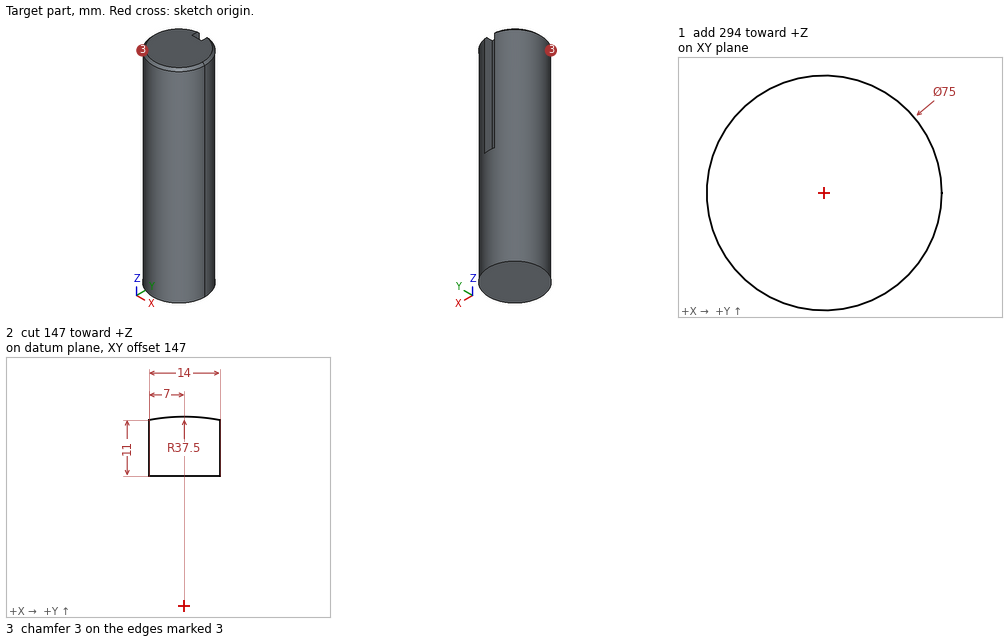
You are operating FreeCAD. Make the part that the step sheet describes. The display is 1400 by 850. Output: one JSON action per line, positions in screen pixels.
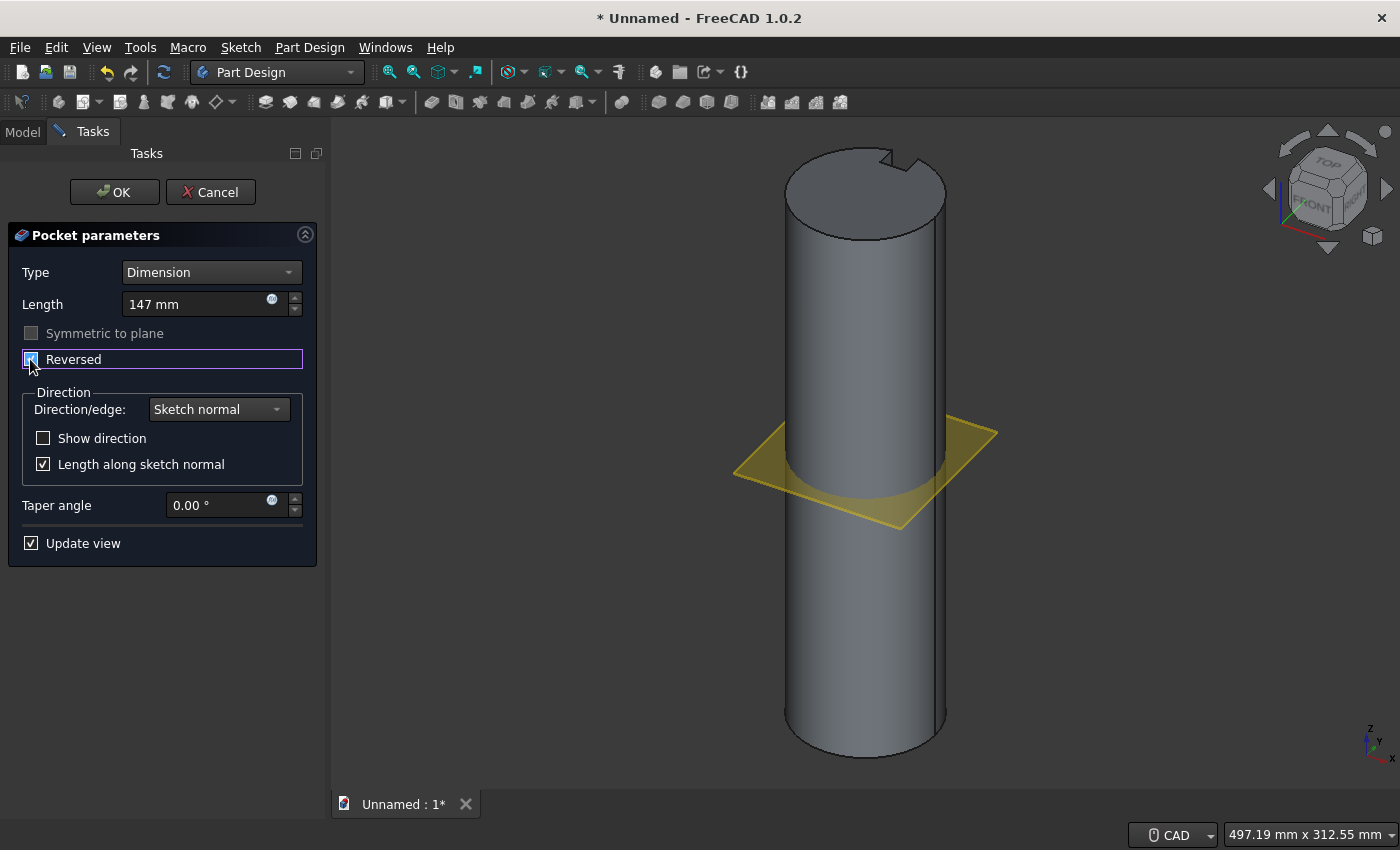
{"action": "left_click", "coordinate": [115, 192]}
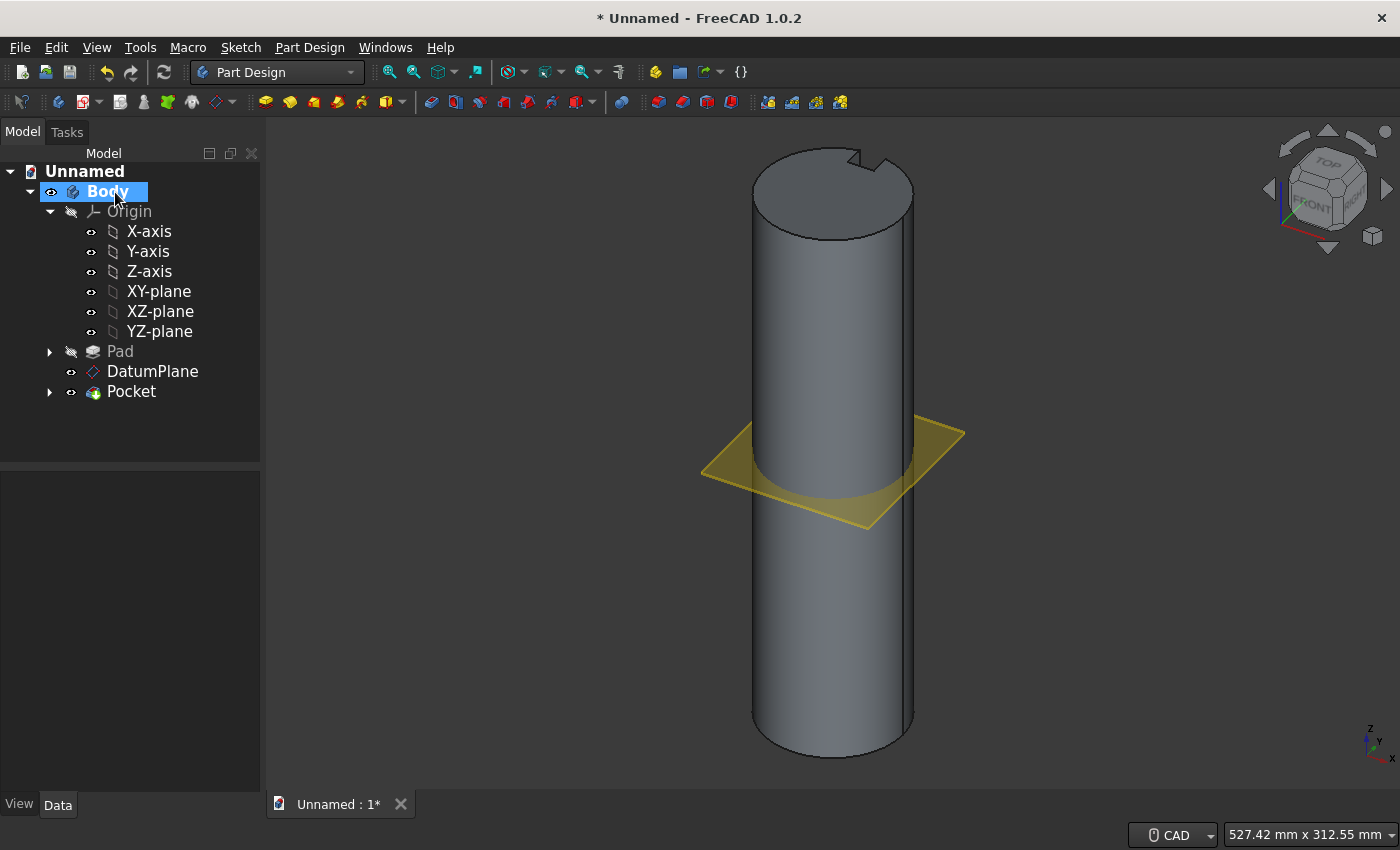
{"action": "left_click", "coordinate": [116, 372]}
{"action": "key", "text": "space"}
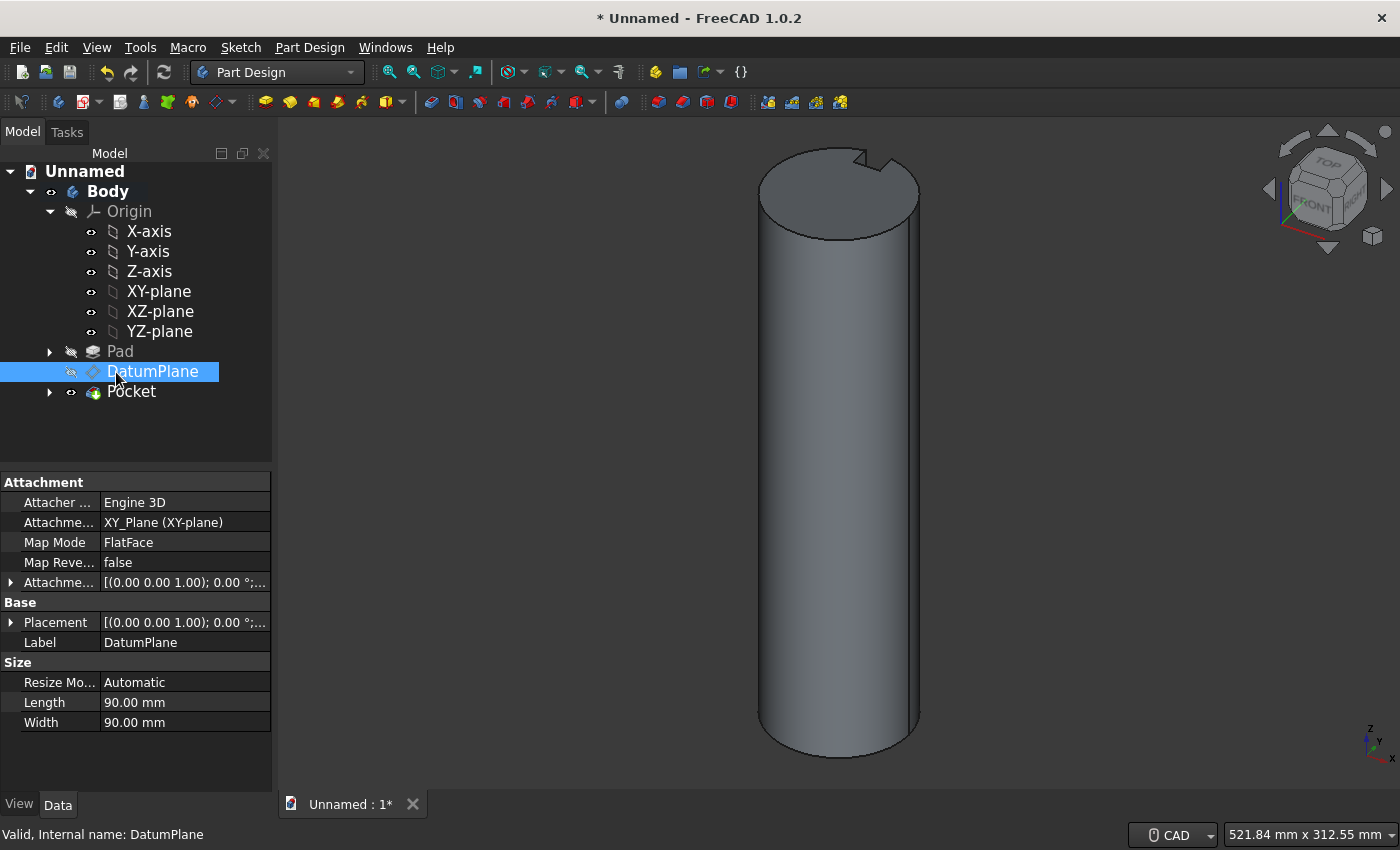
{"action": "left_click", "coordinate": [763, 209]}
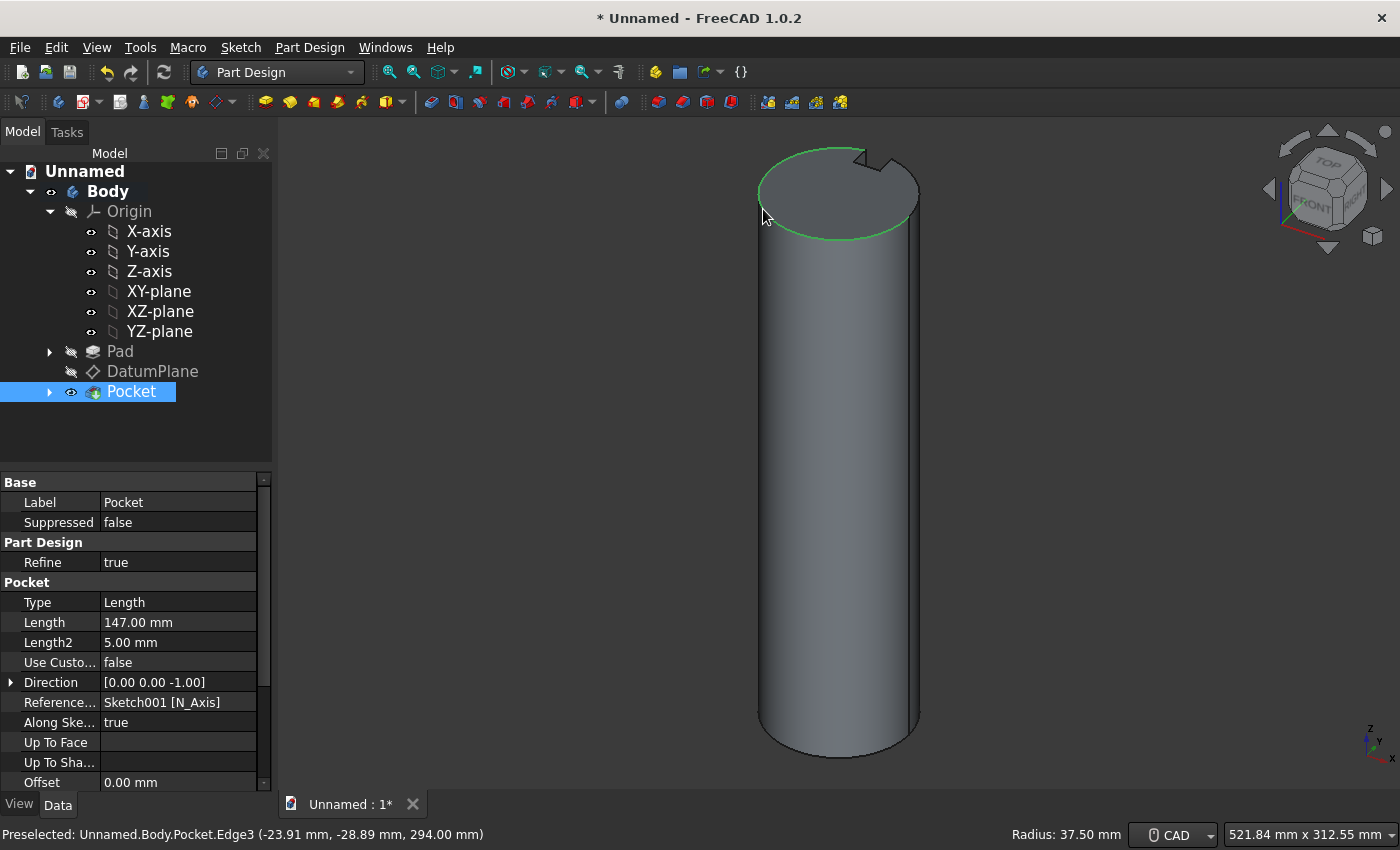
{"action": "left_click", "coordinate": [684, 102]}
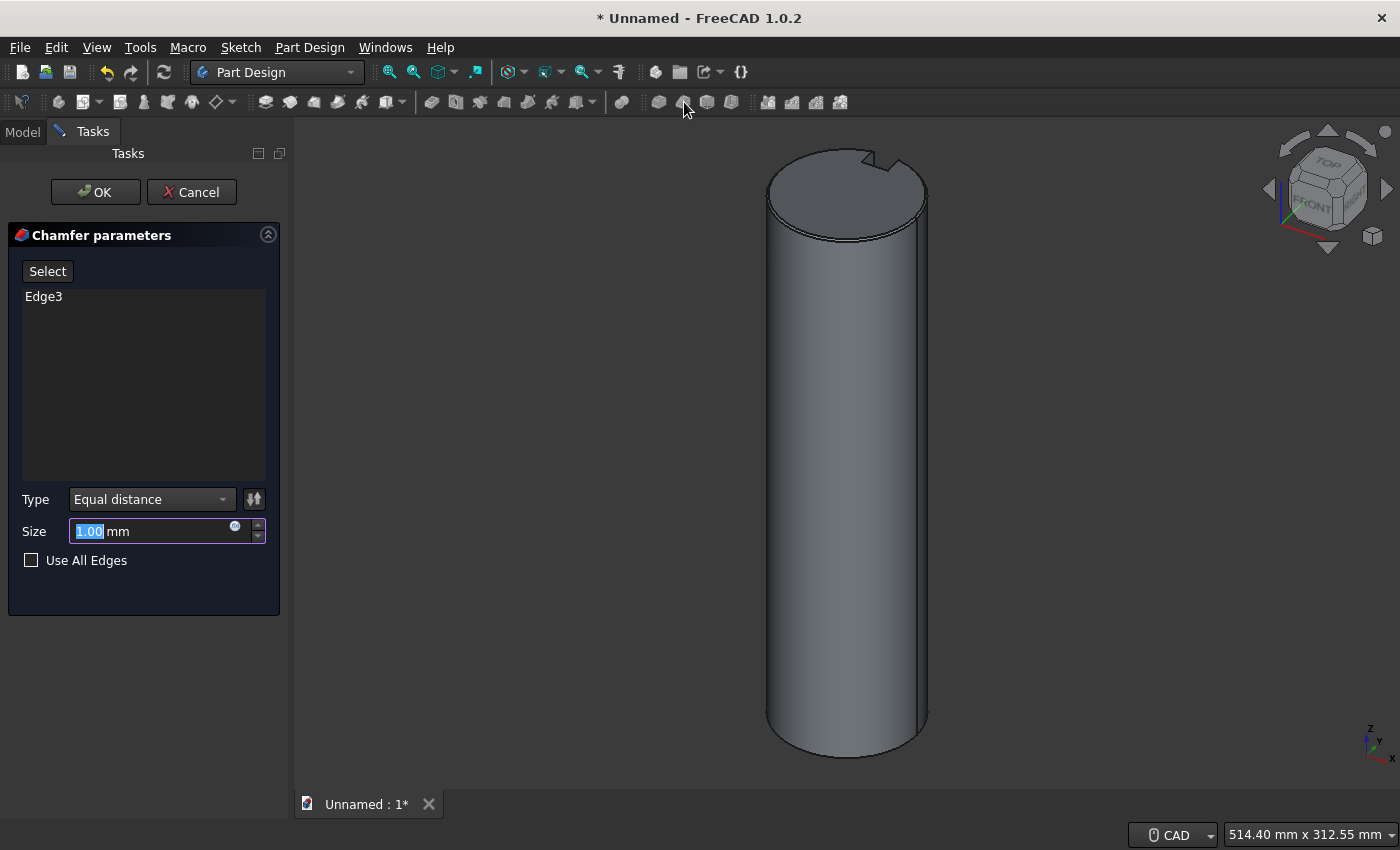
{"action": "type", "text": "3"}
{"action": "key", "text": "Tab"}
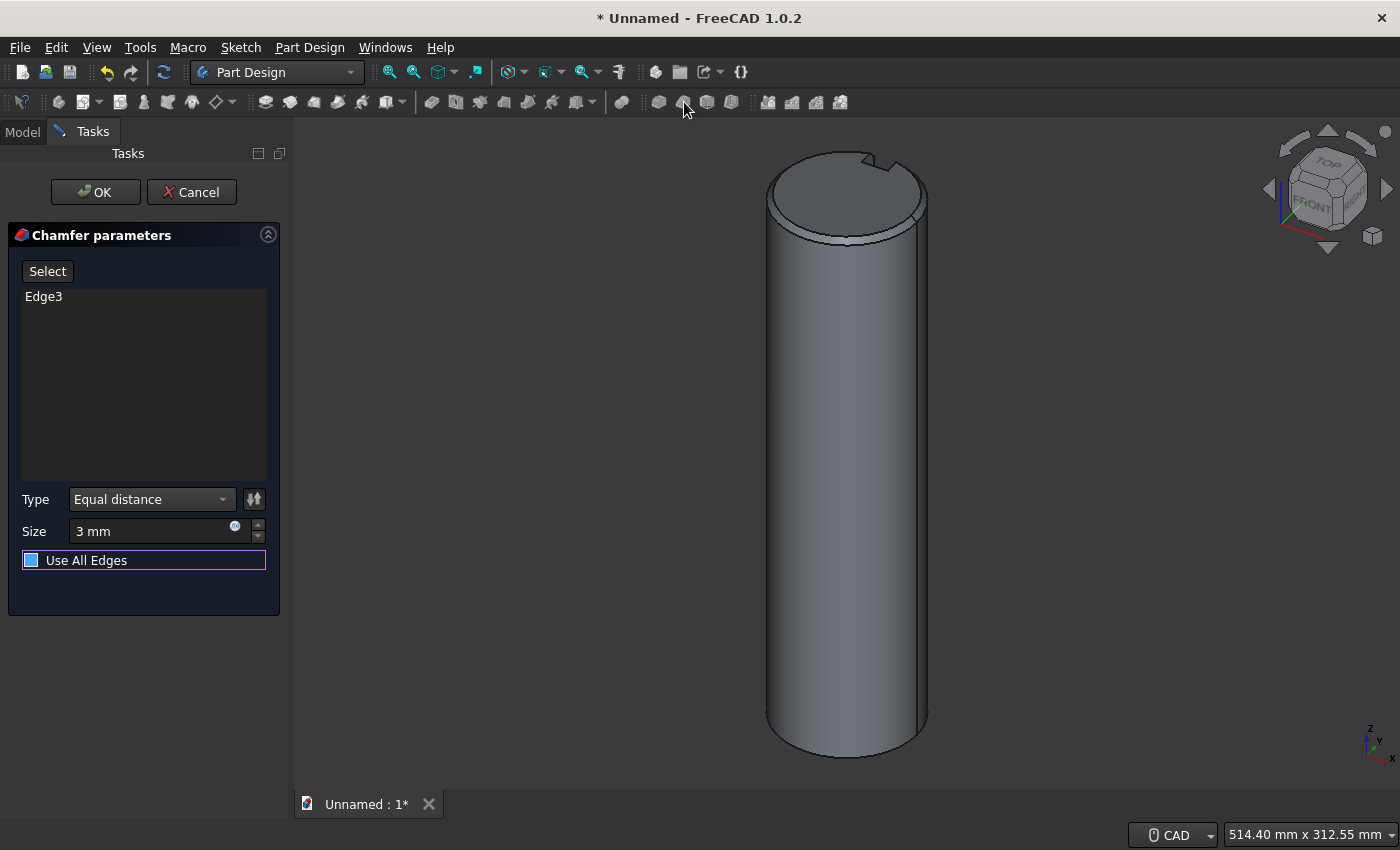
{"action": "left_click", "coordinate": [96, 192]}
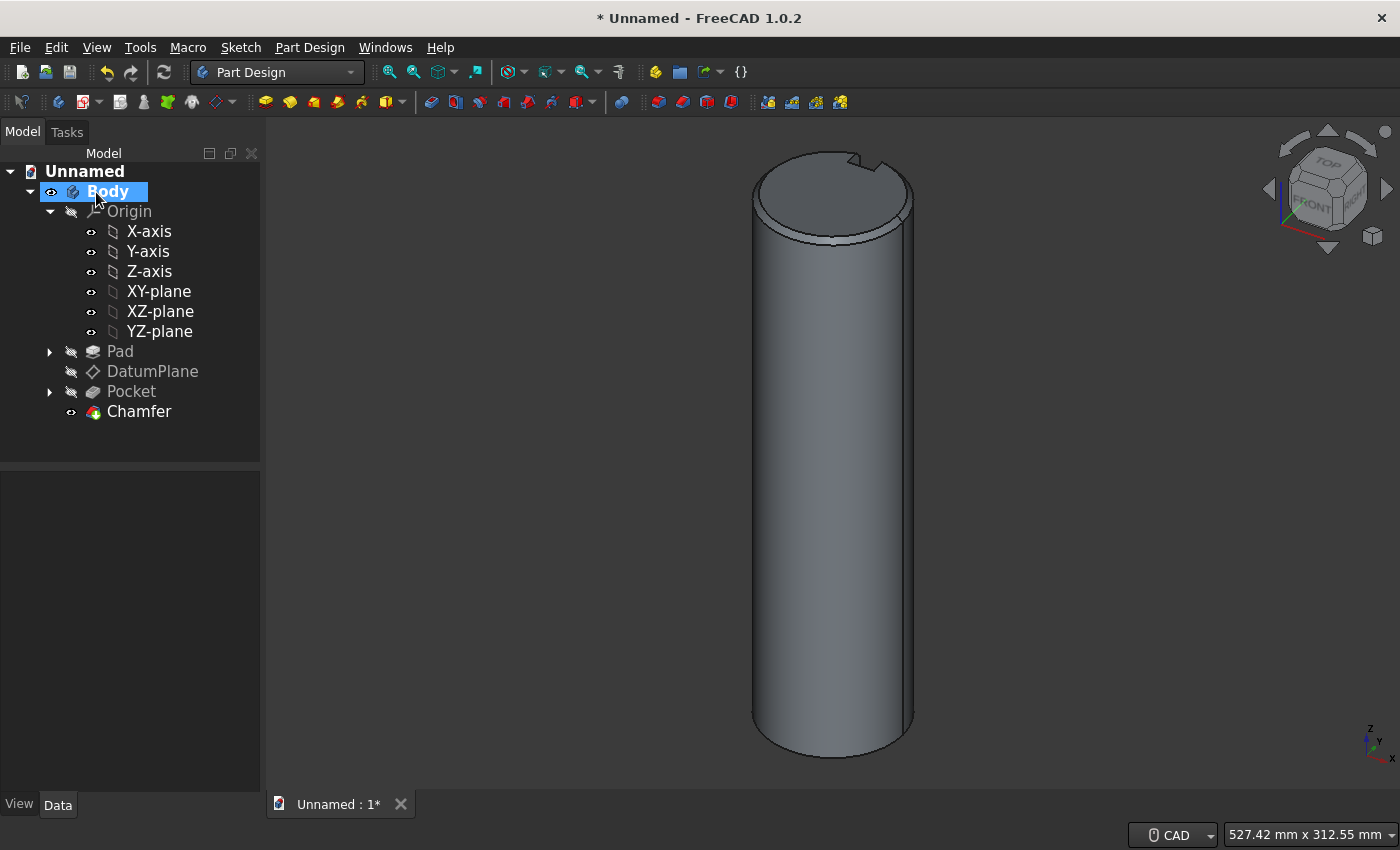
{"action": "key", "text": "0"}